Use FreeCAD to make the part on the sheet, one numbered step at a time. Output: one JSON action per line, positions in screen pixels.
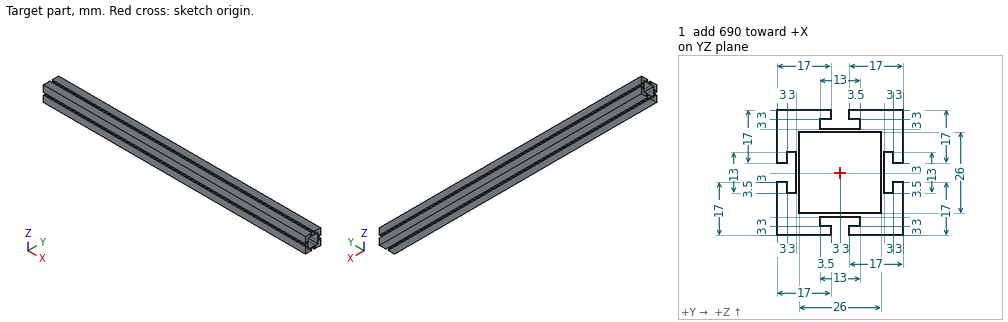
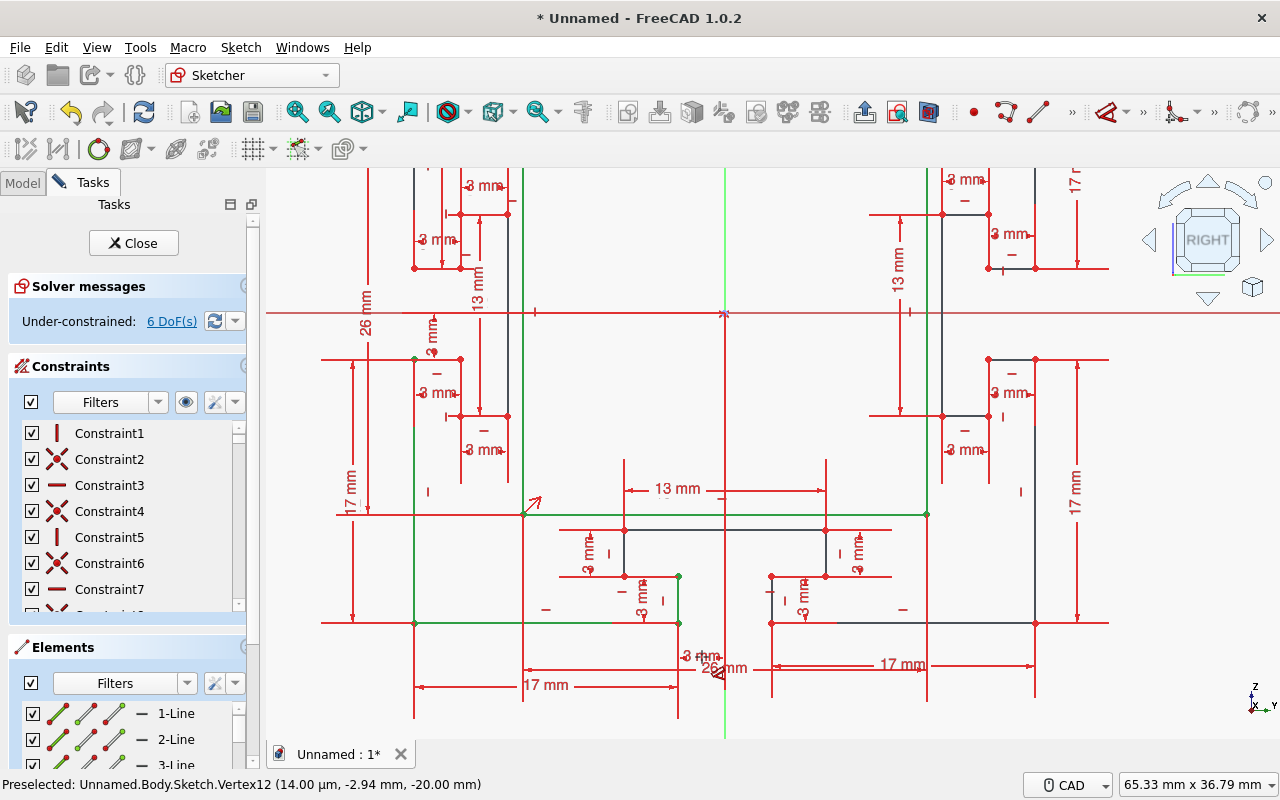
{"action": "left_click", "coordinate": [772, 577]}
{"action": "left_click", "coordinate": [748, 279]}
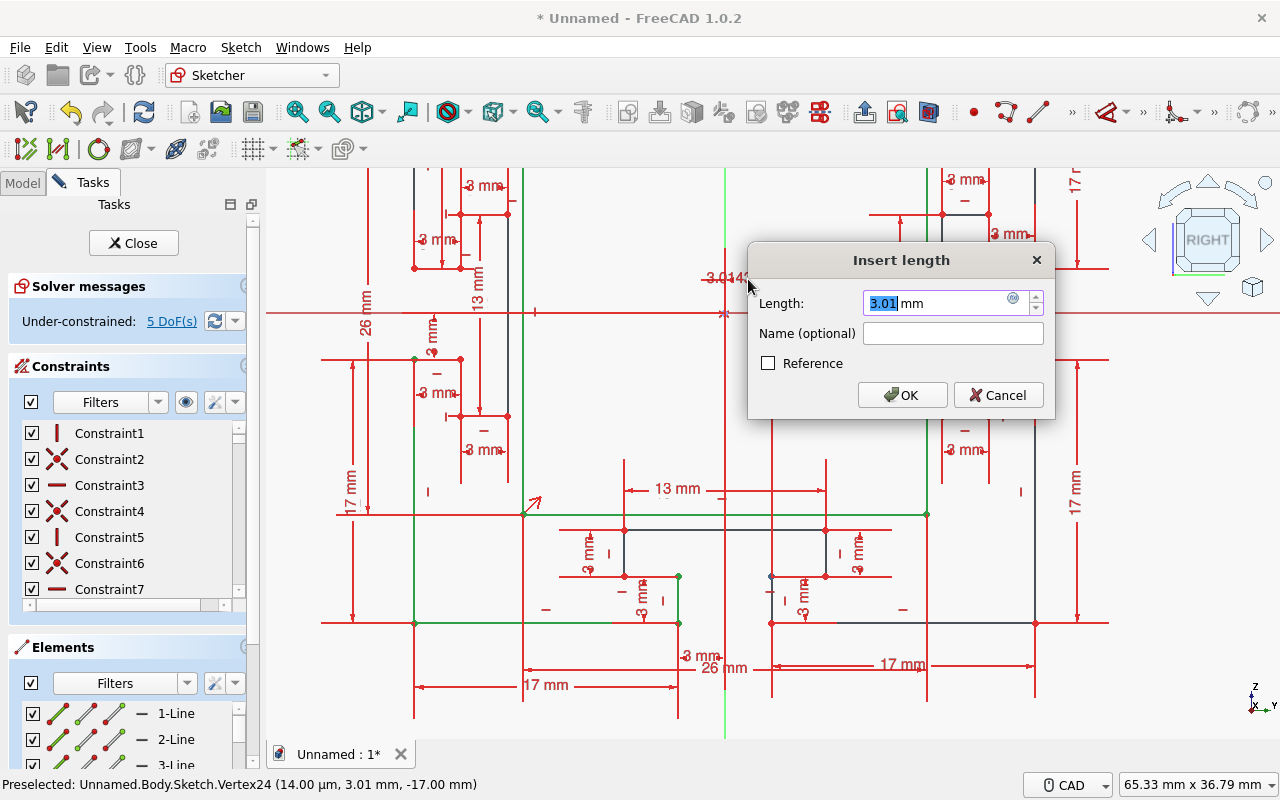
{"action": "type", "text": "3"}
{"action": "key", "text": "Return"}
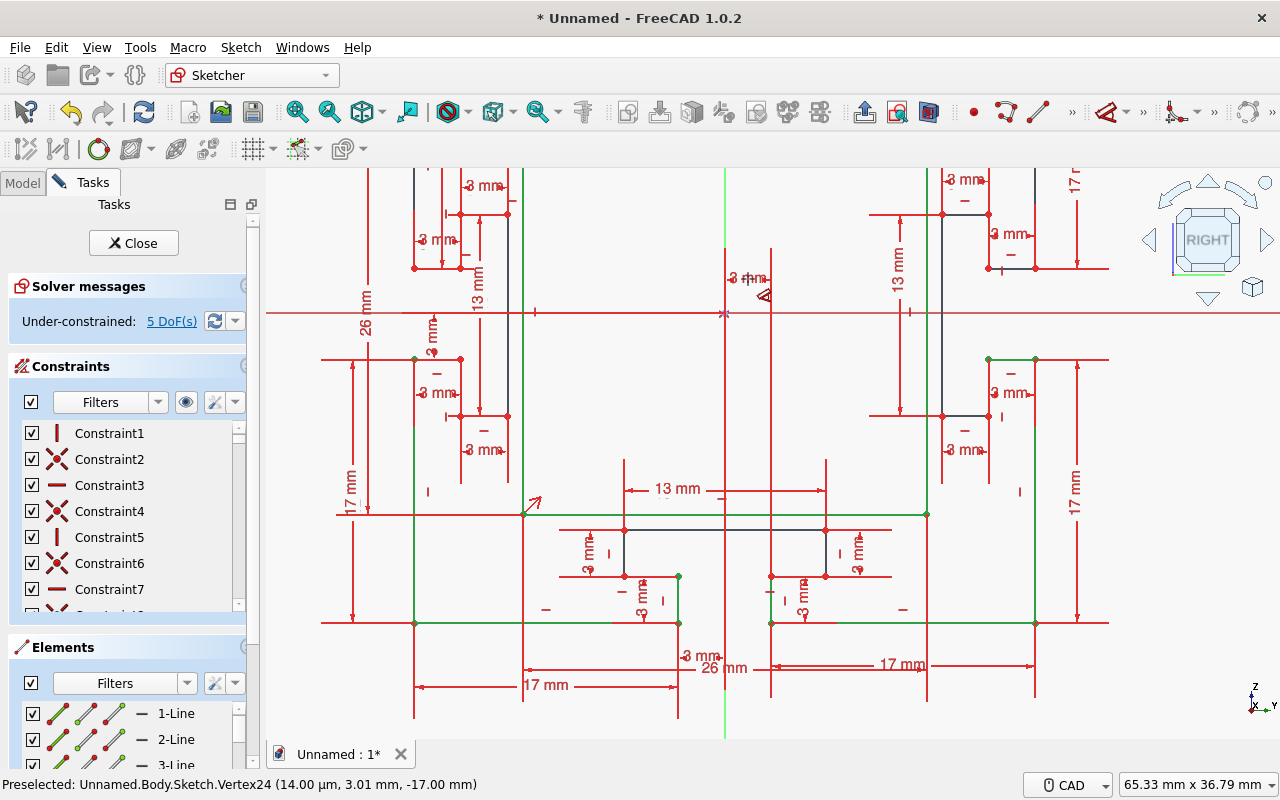
{"action": "left_click", "coordinate": [989, 269]}
{"action": "left_click", "coordinate": [1023, 291]}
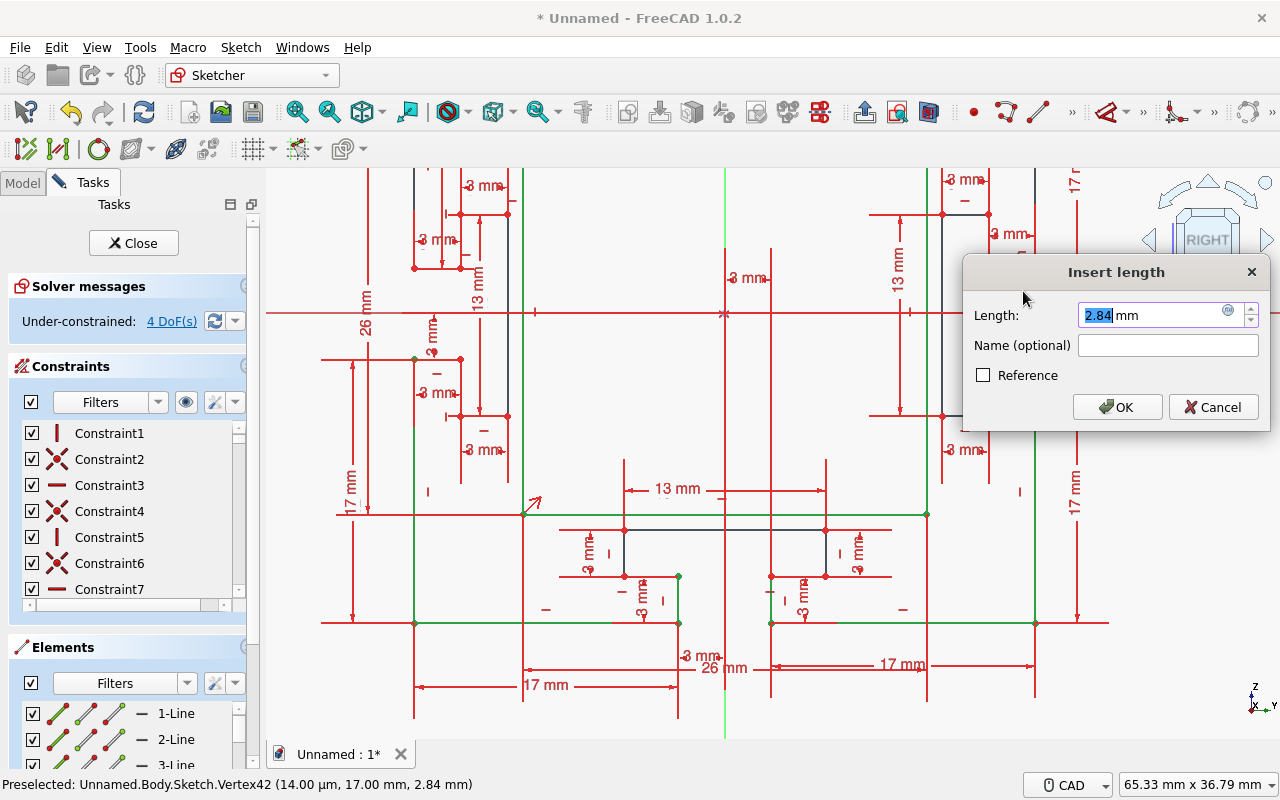
{"action": "type", "text": "3"}
{"action": "key", "text": "Return"}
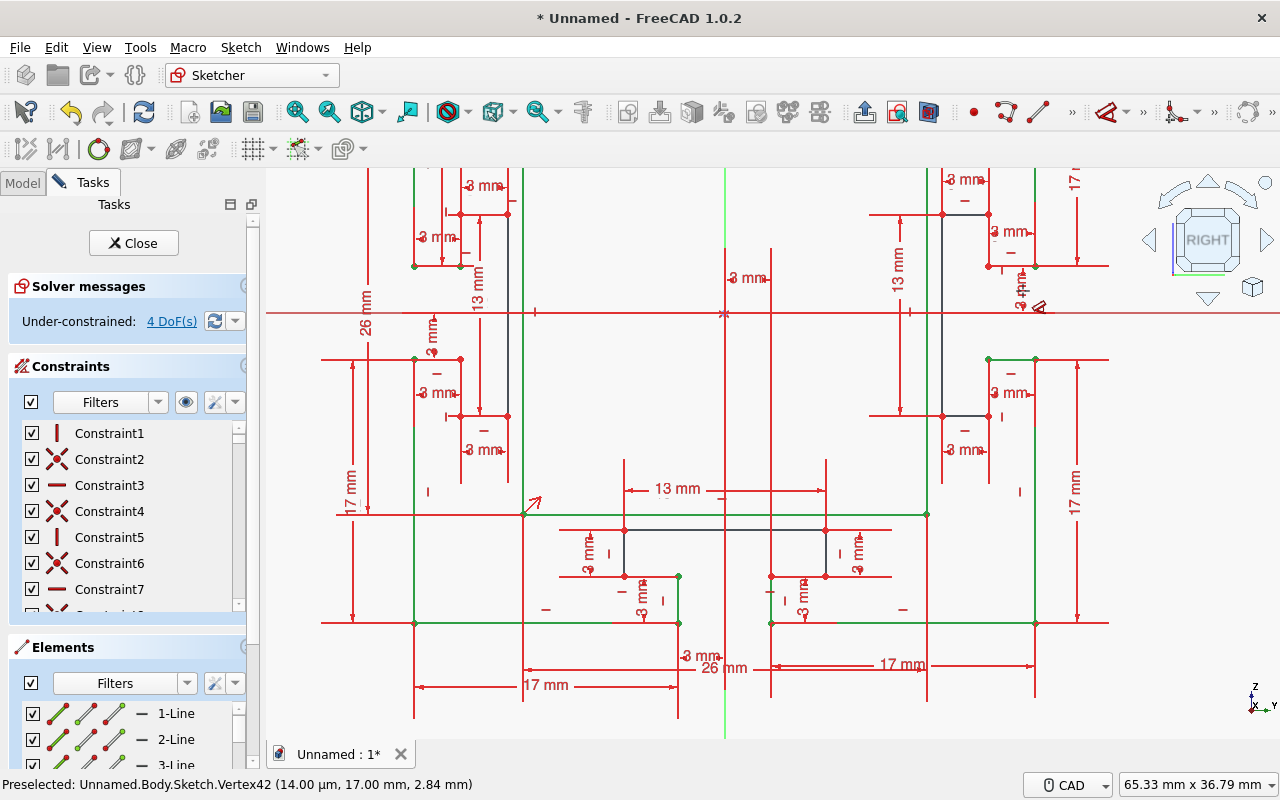
{"action": "left_click", "coordinate": [461, 399]}
{"action": "left_click", "coordinate": [379, 375]}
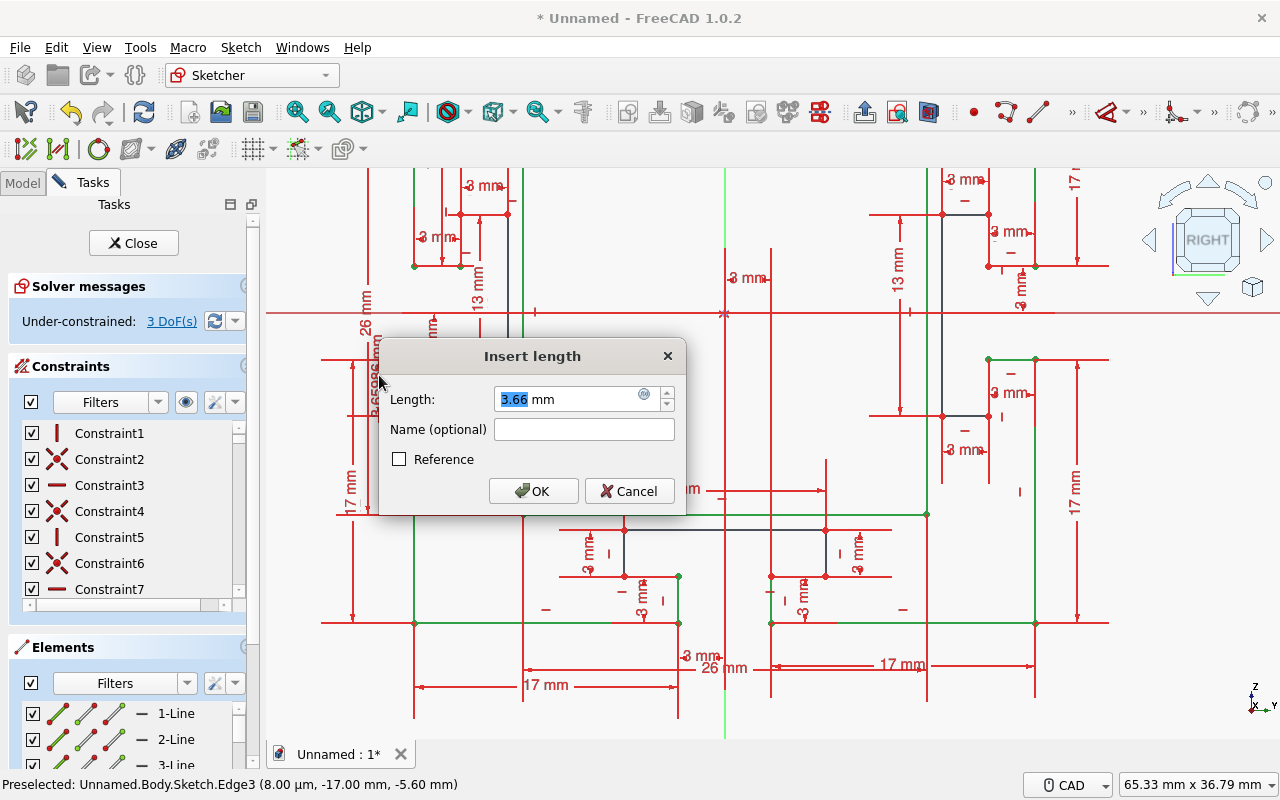
{"action": "type", "text": "3.5"}
{"action": "key", "text": "Return"}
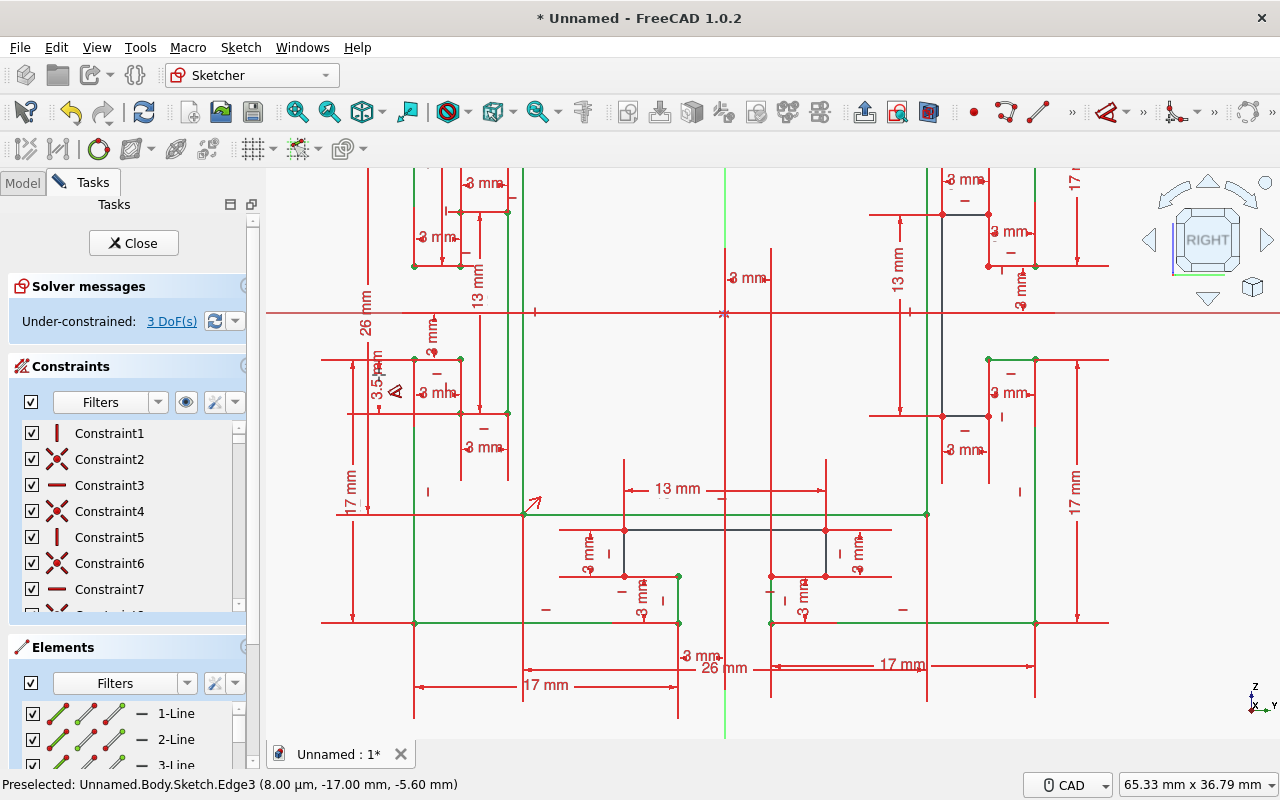
{"action": "left_click", "coordinate": [662, 577]}
{"action": "left_click", "coordinate": [651, 683]}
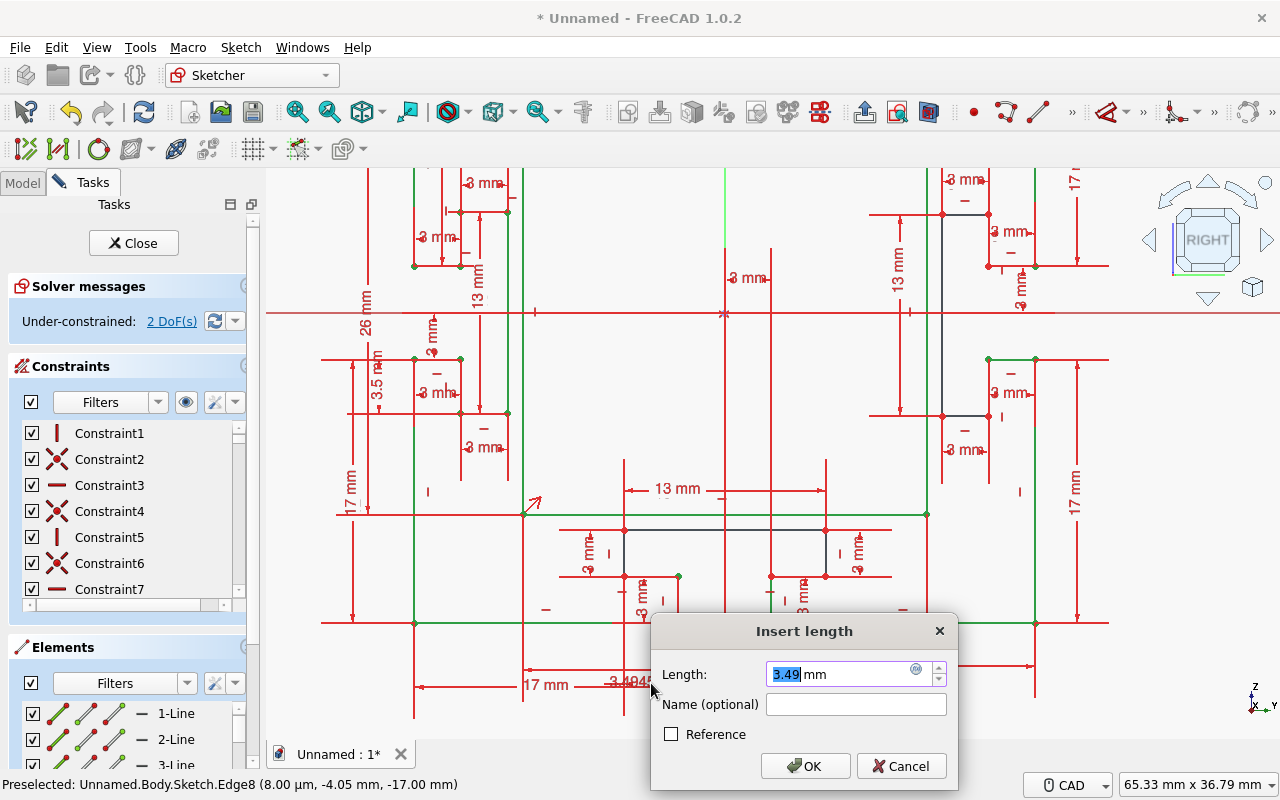
{"action": "type", "text": "3.5"}
{"action": "key", "text": "Return"}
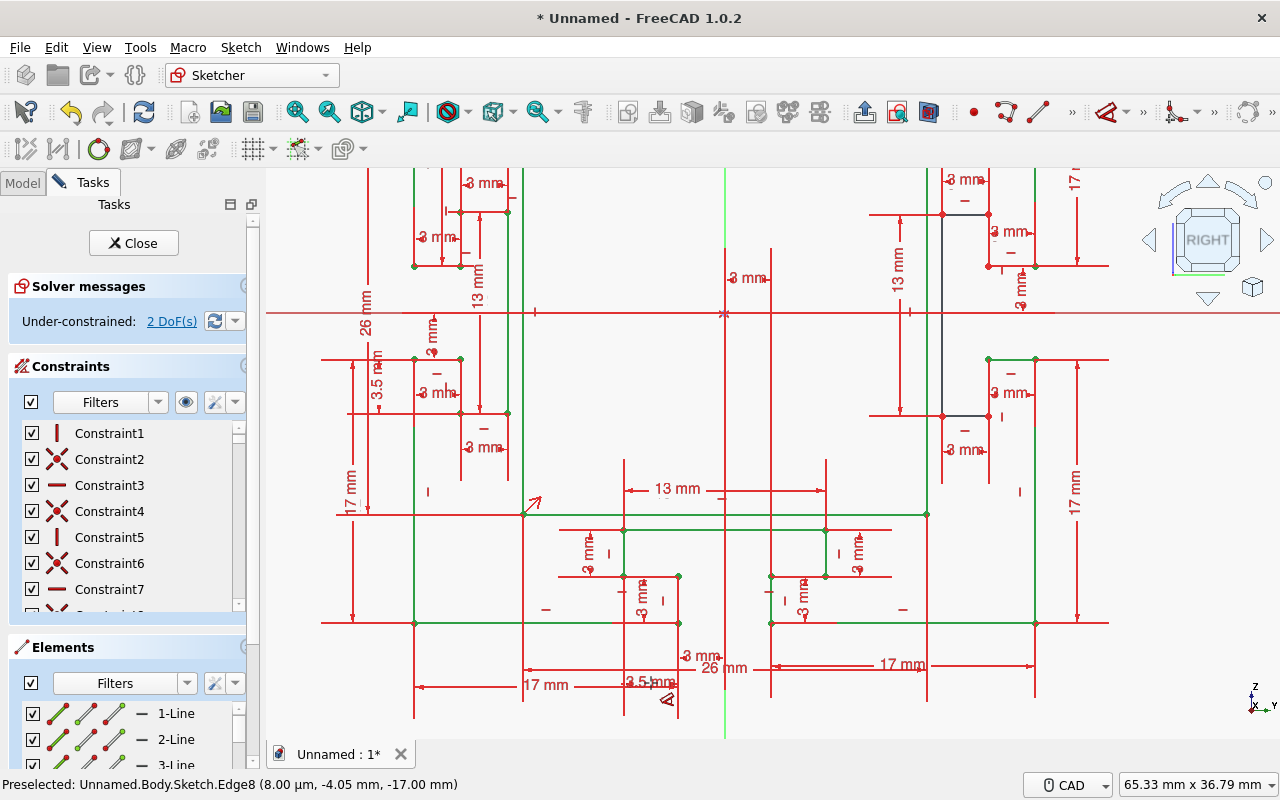
{"action": "left_click", "coordinate": [989, 377]}
{"action": "left_click", "coordinate": [1071, 375]}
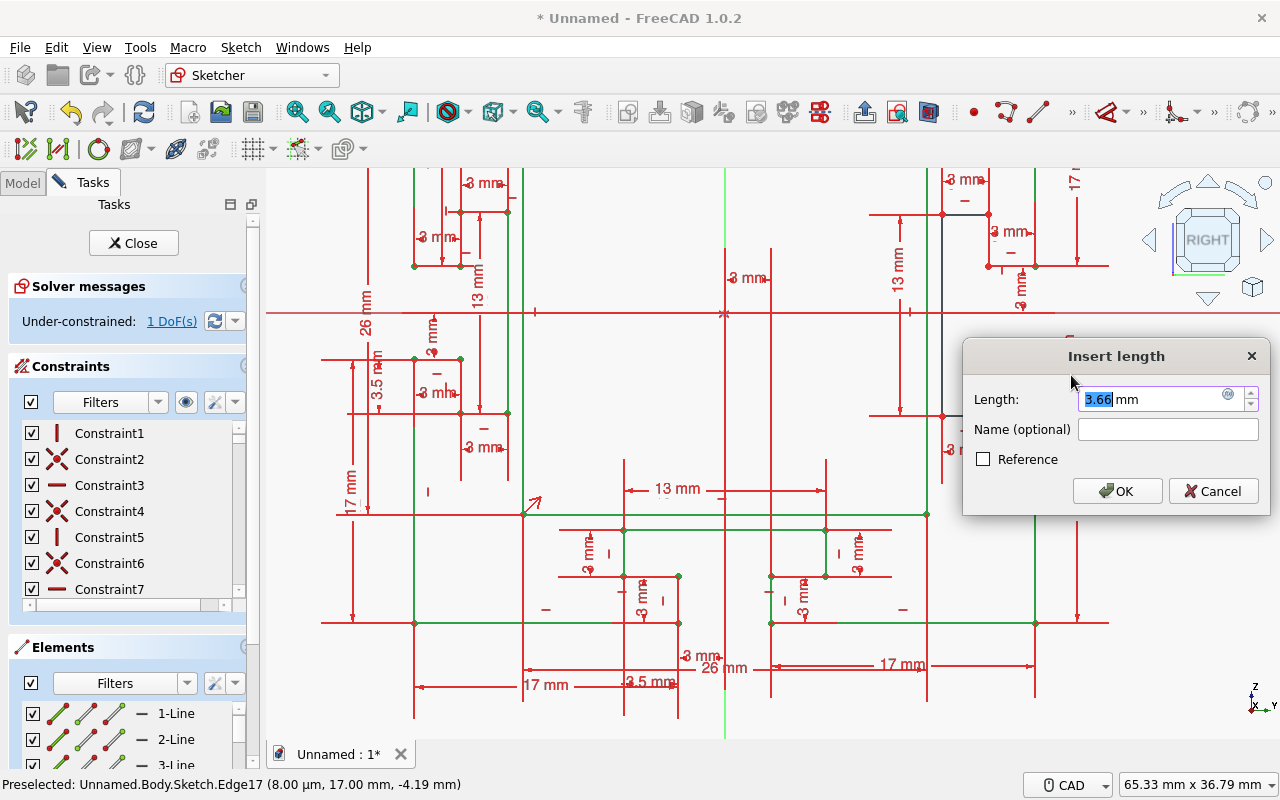
{"action": "type", "text": "3.5"}
{"action": "key", "text": "Return"}